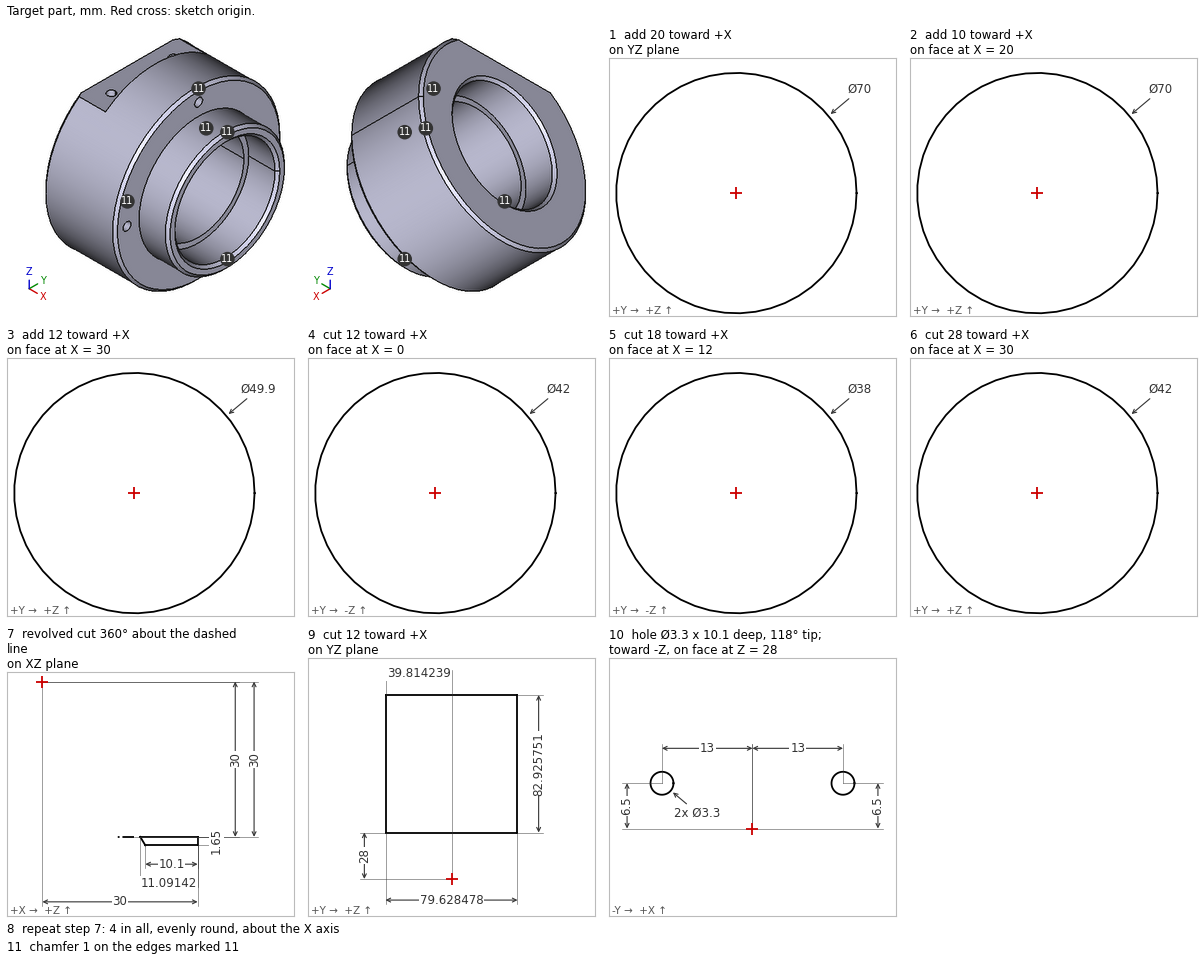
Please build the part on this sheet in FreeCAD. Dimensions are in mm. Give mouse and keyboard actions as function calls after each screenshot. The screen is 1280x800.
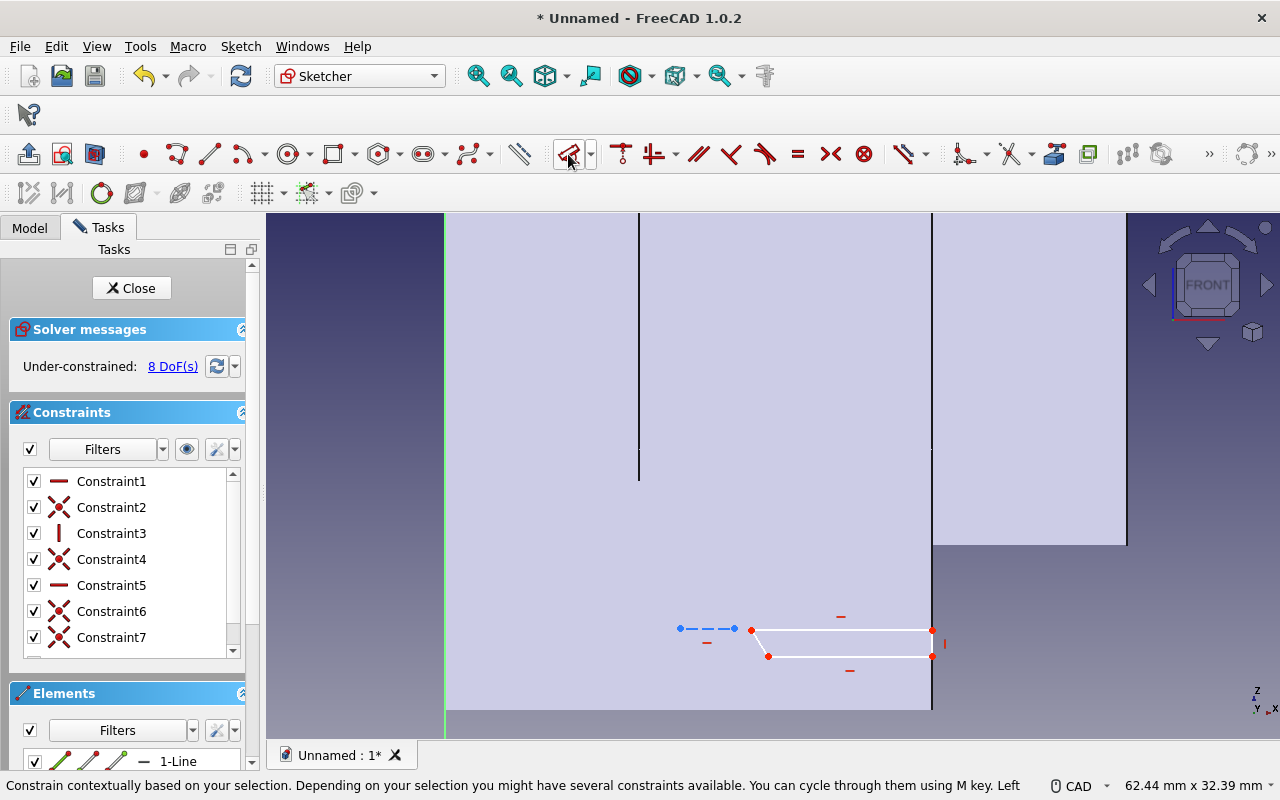
click(752, 630)
click(411, 436)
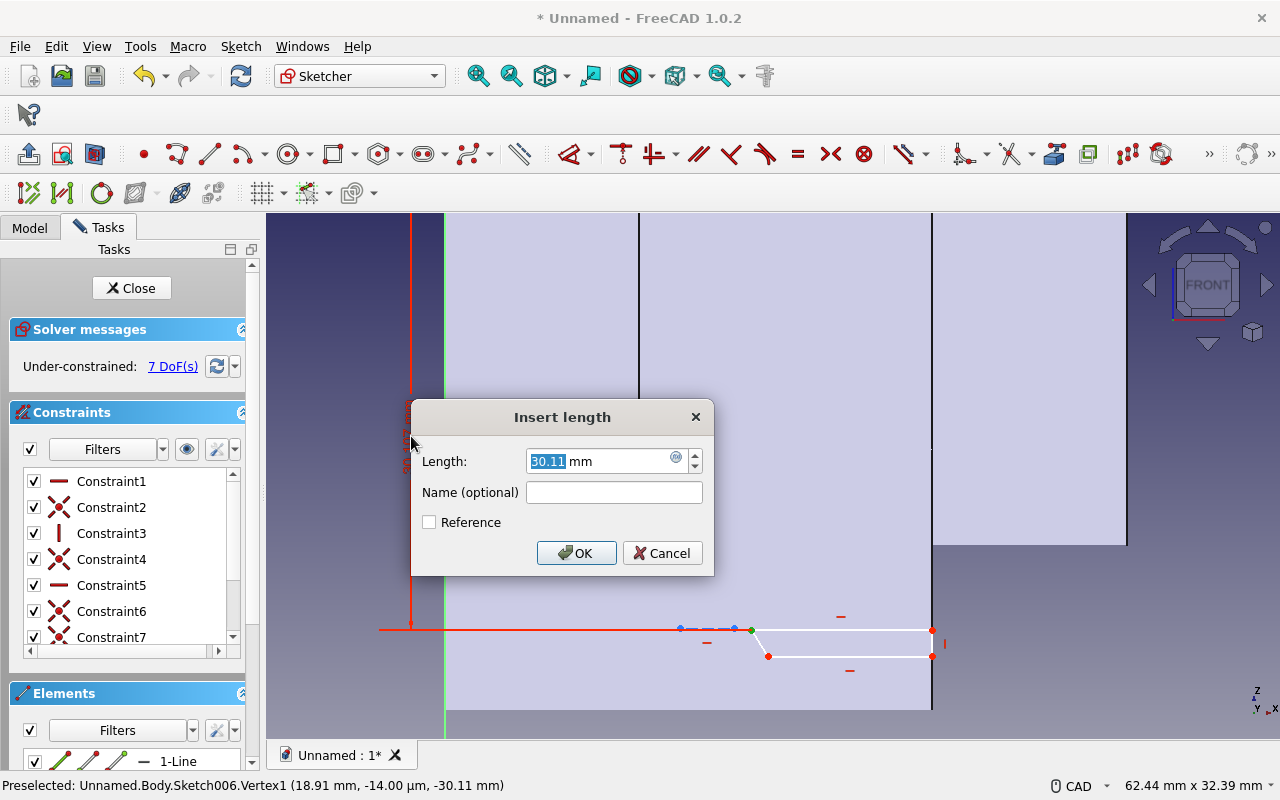
text(30)
key(Return)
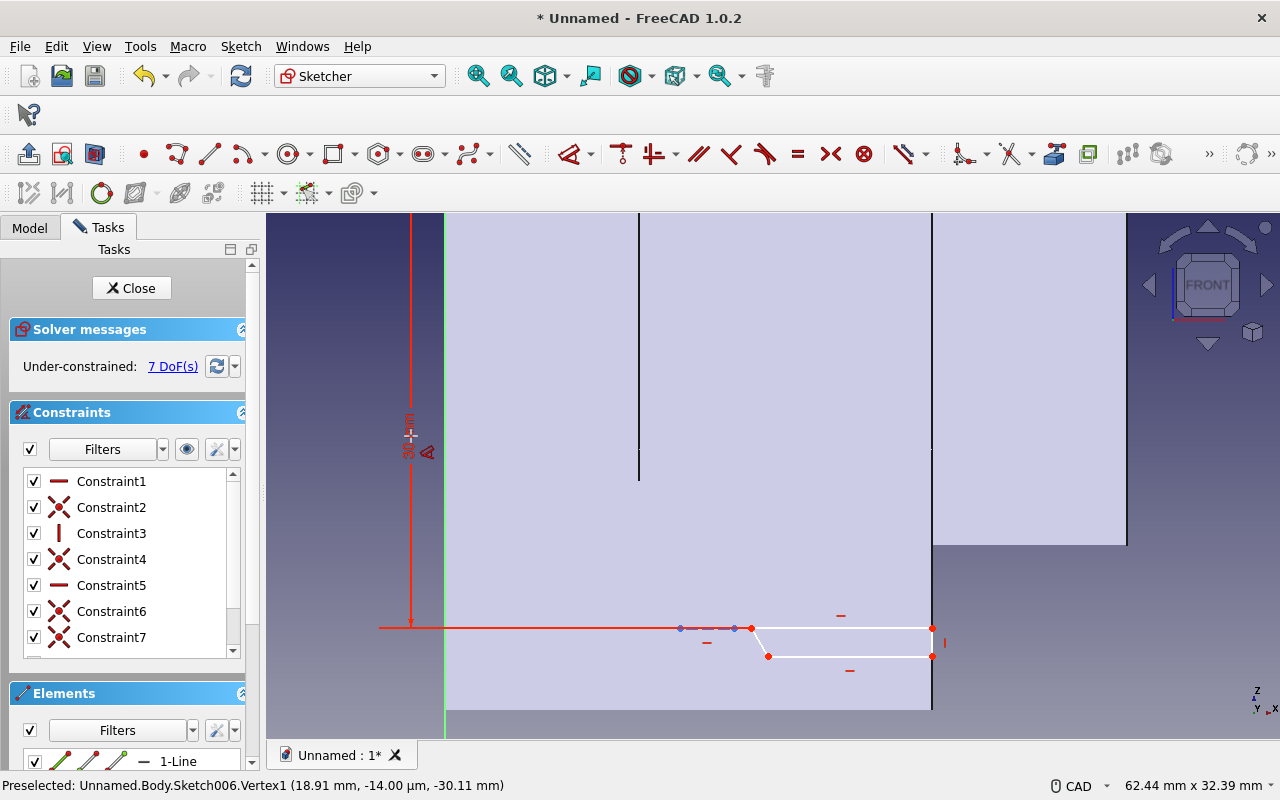
click(932, 628)
click(688, 662)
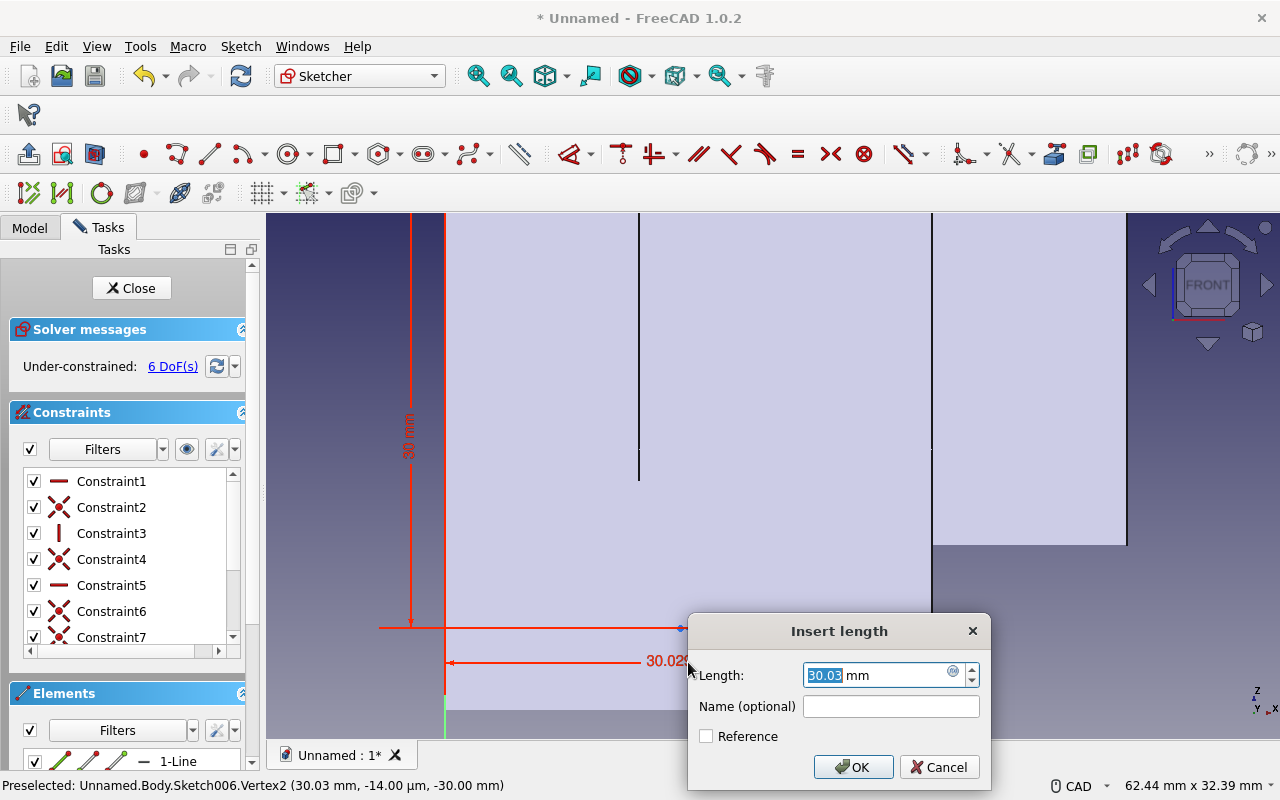
text(30)
key(Return)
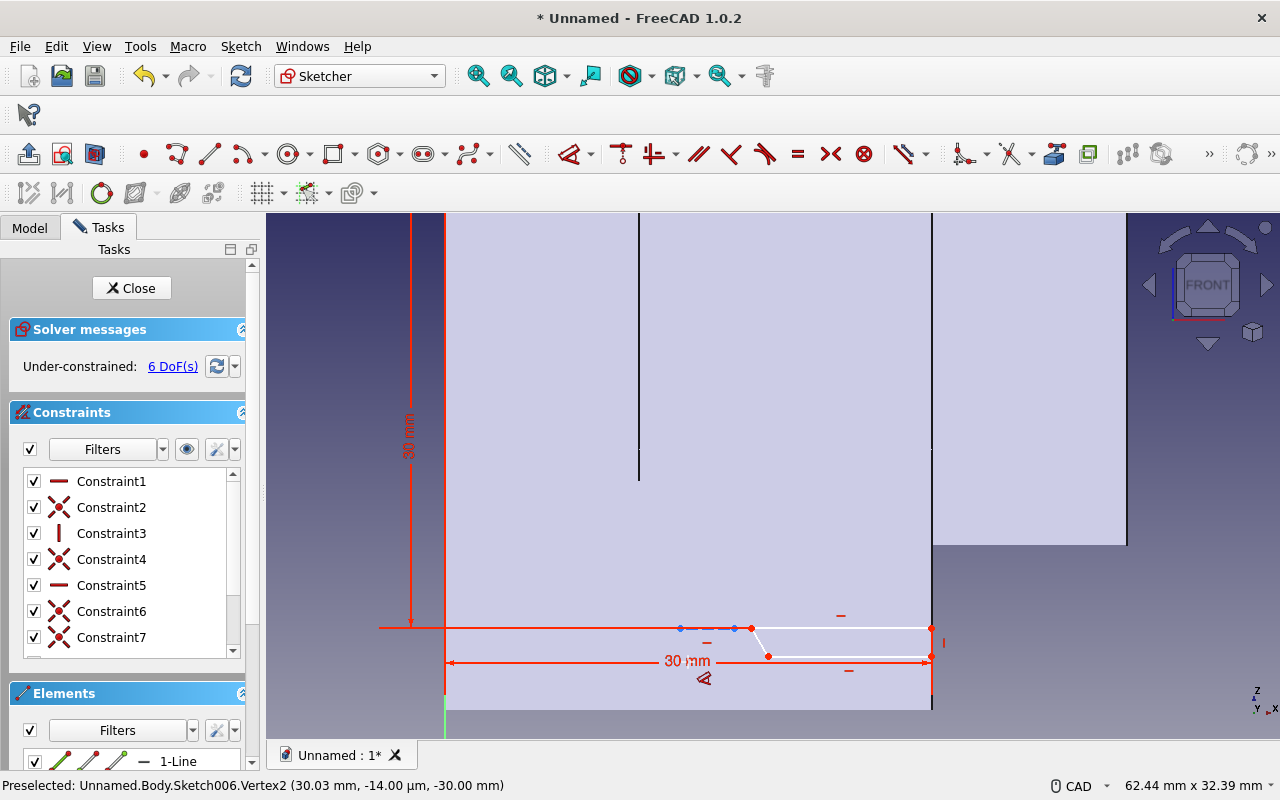
click(734, 629)
click(411, 346)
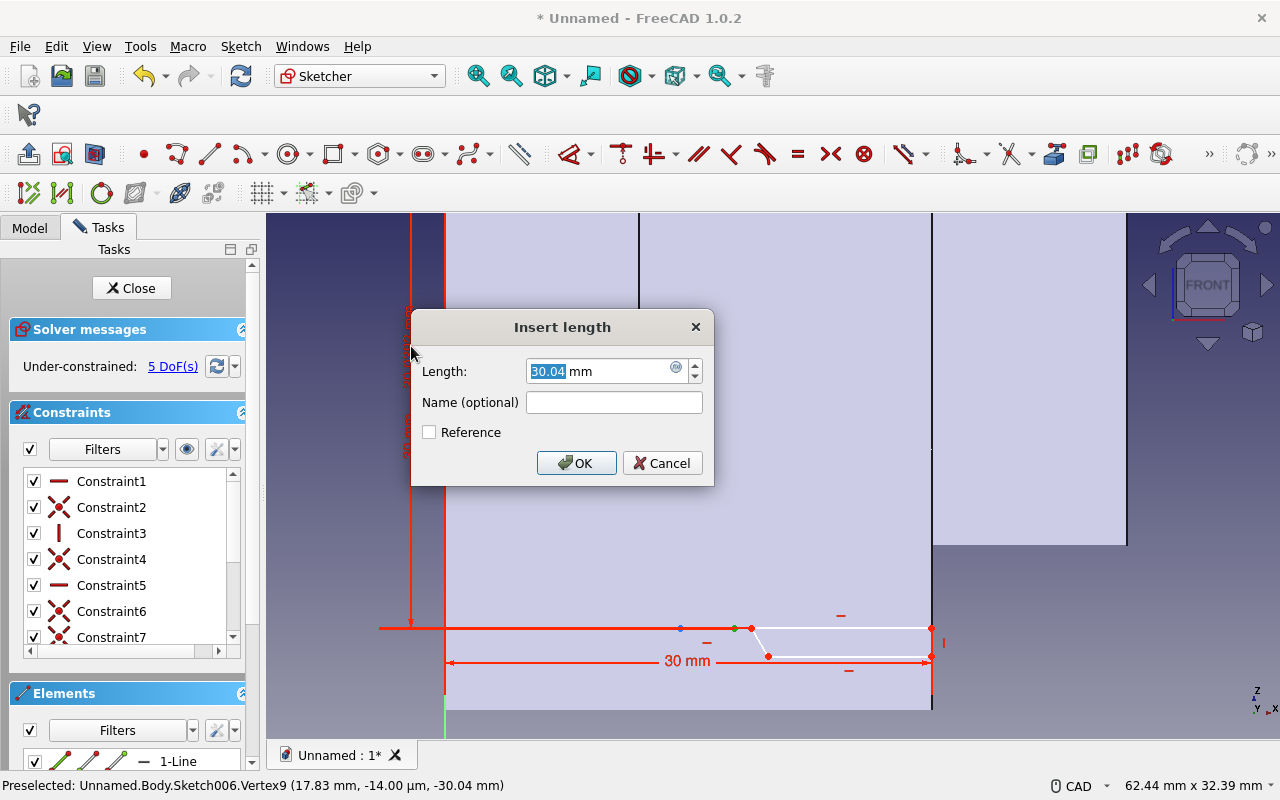
text(30)
key(Return)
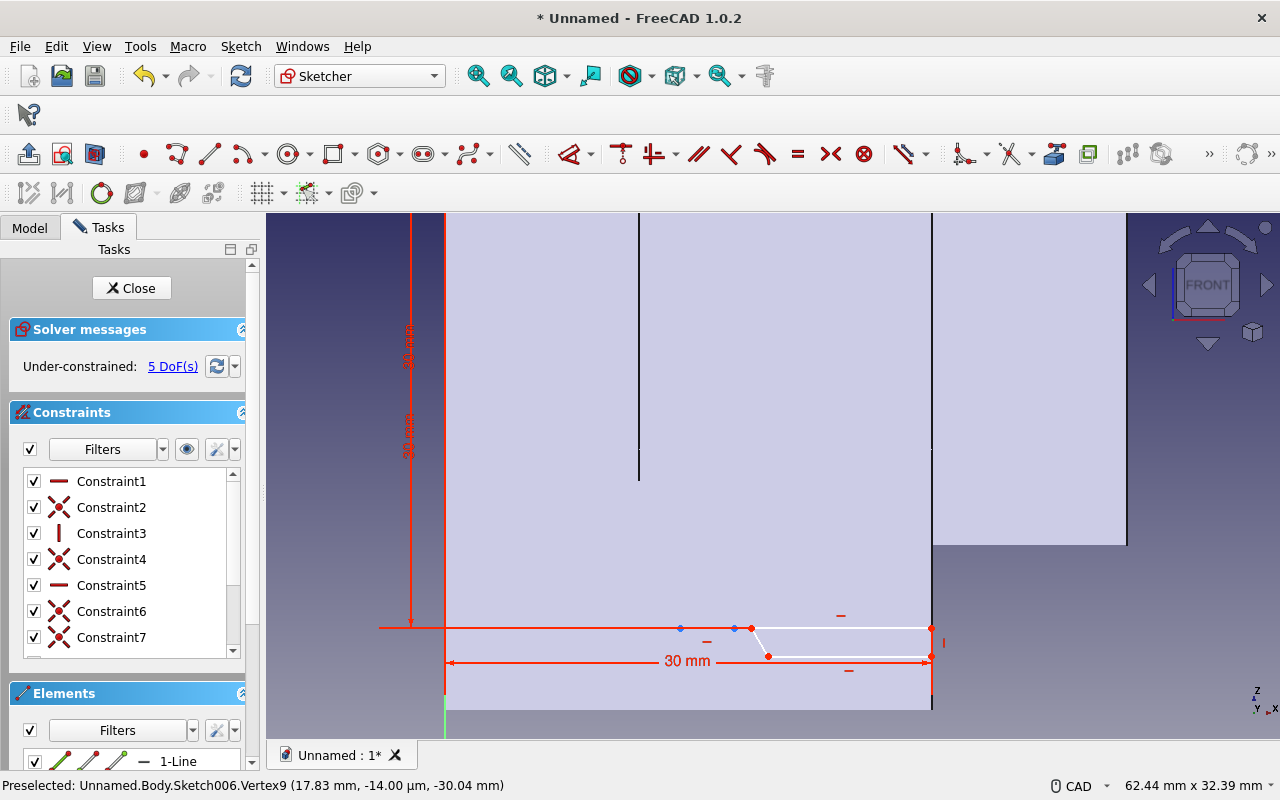
scroll(932, 640, up, 2)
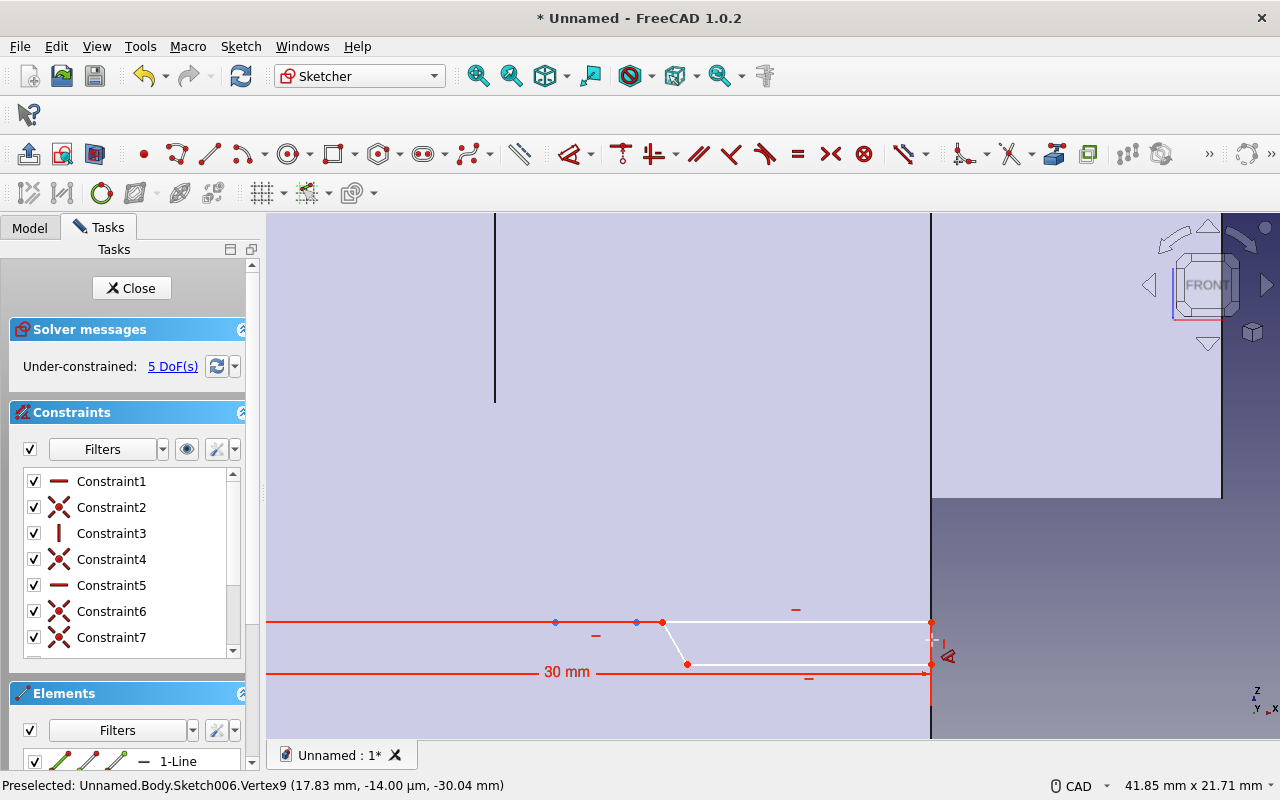
click(931, 639)
click(965, 644)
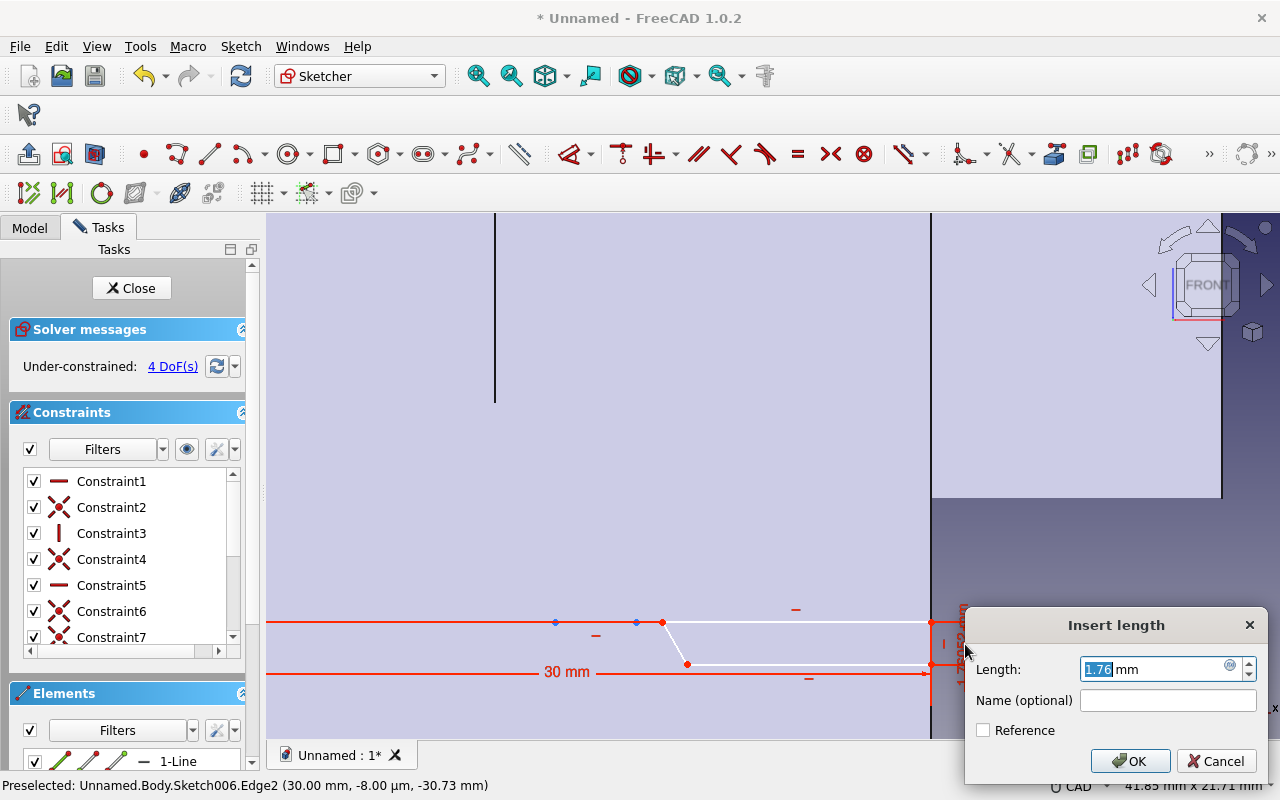
text(1.65)
key(Return)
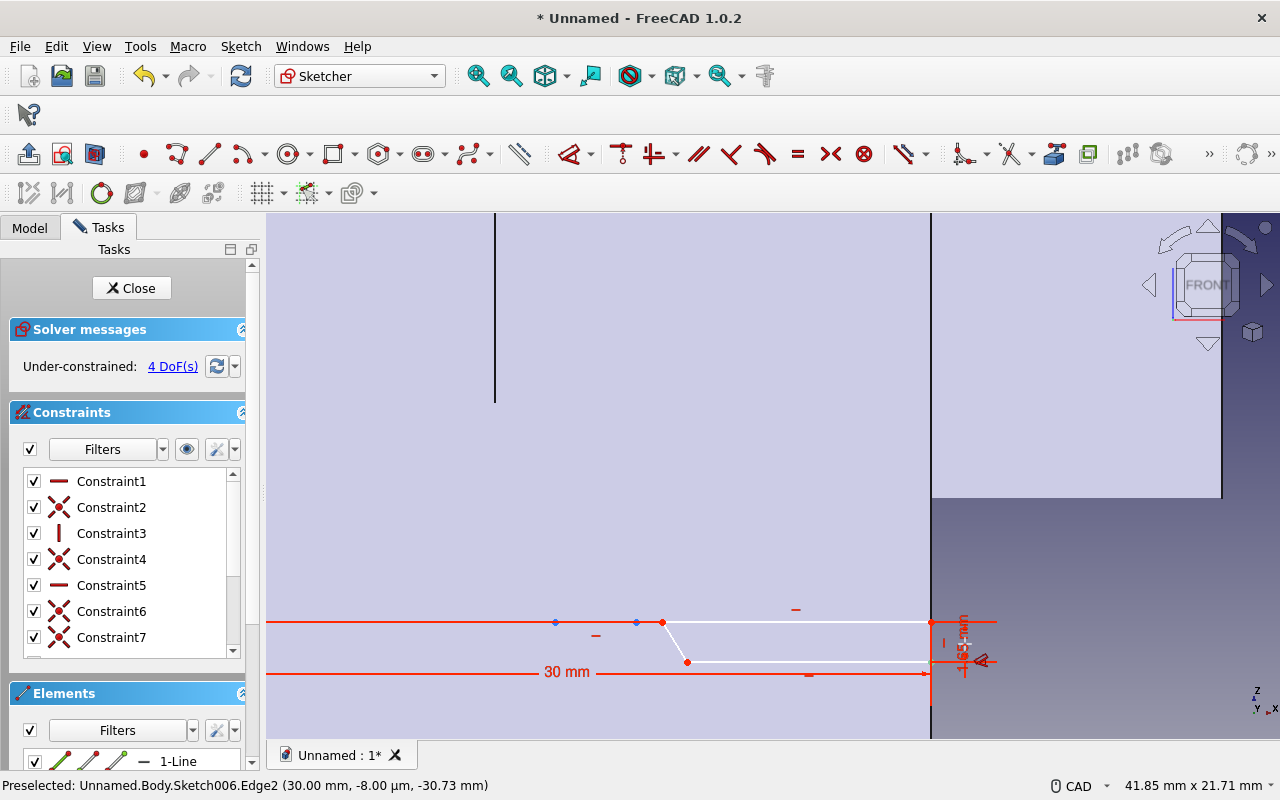
click(858, 662)
click(809, 696)